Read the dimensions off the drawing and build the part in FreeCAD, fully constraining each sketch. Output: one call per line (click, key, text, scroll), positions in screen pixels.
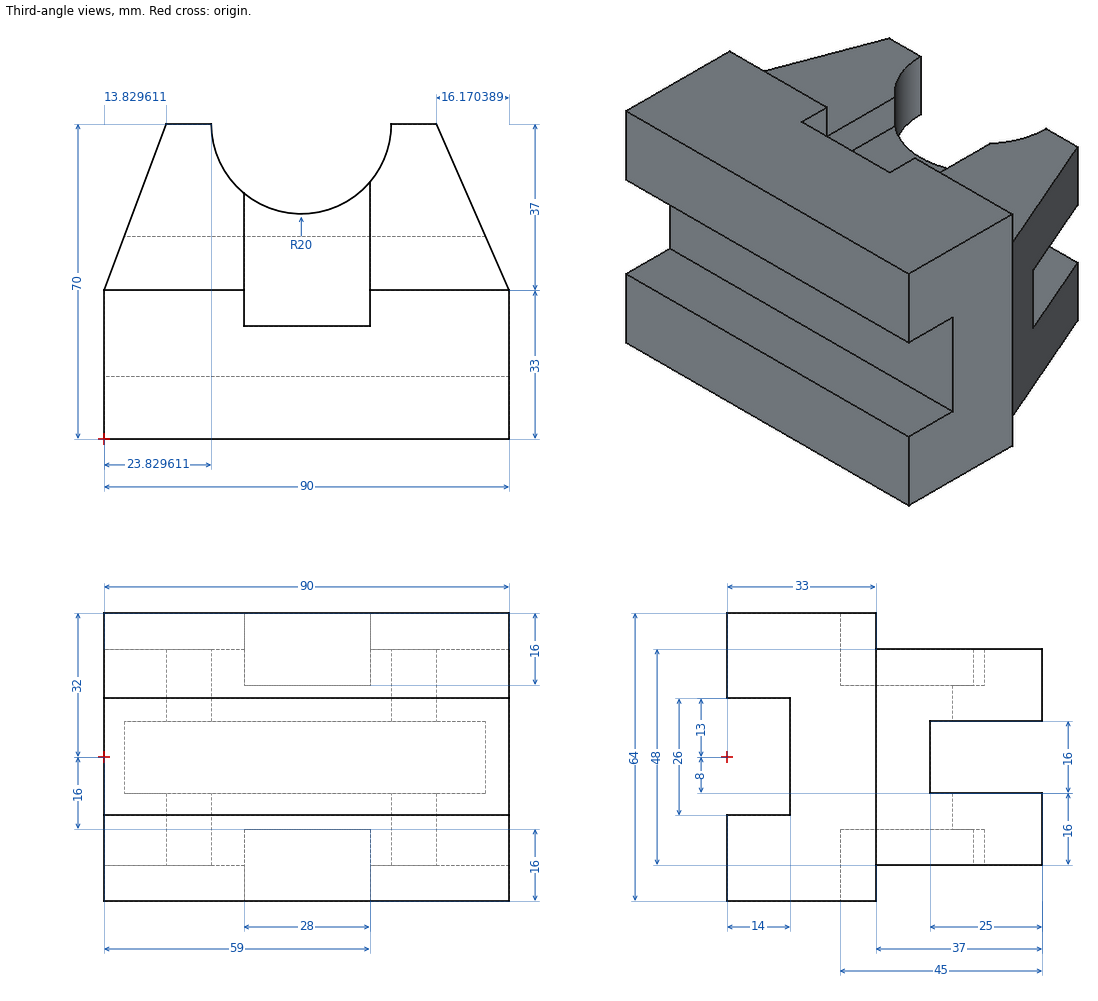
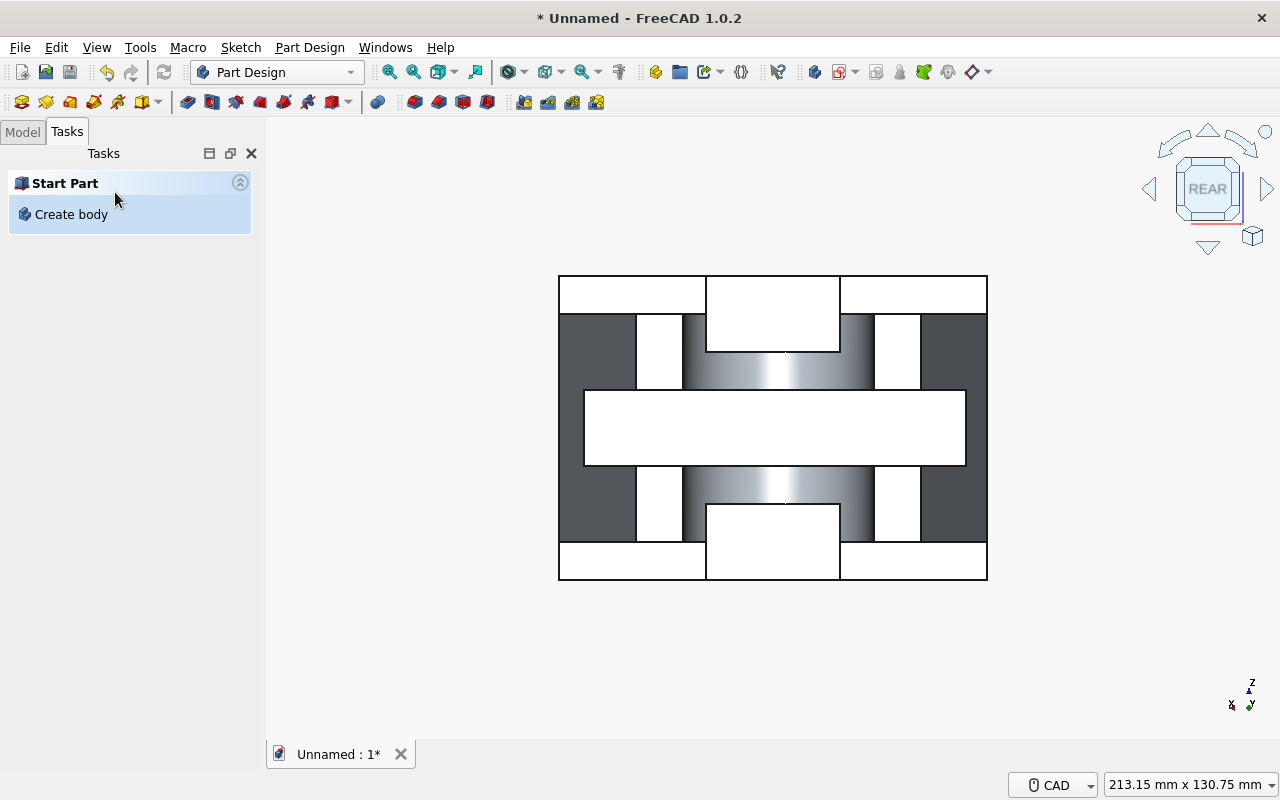
key(0)